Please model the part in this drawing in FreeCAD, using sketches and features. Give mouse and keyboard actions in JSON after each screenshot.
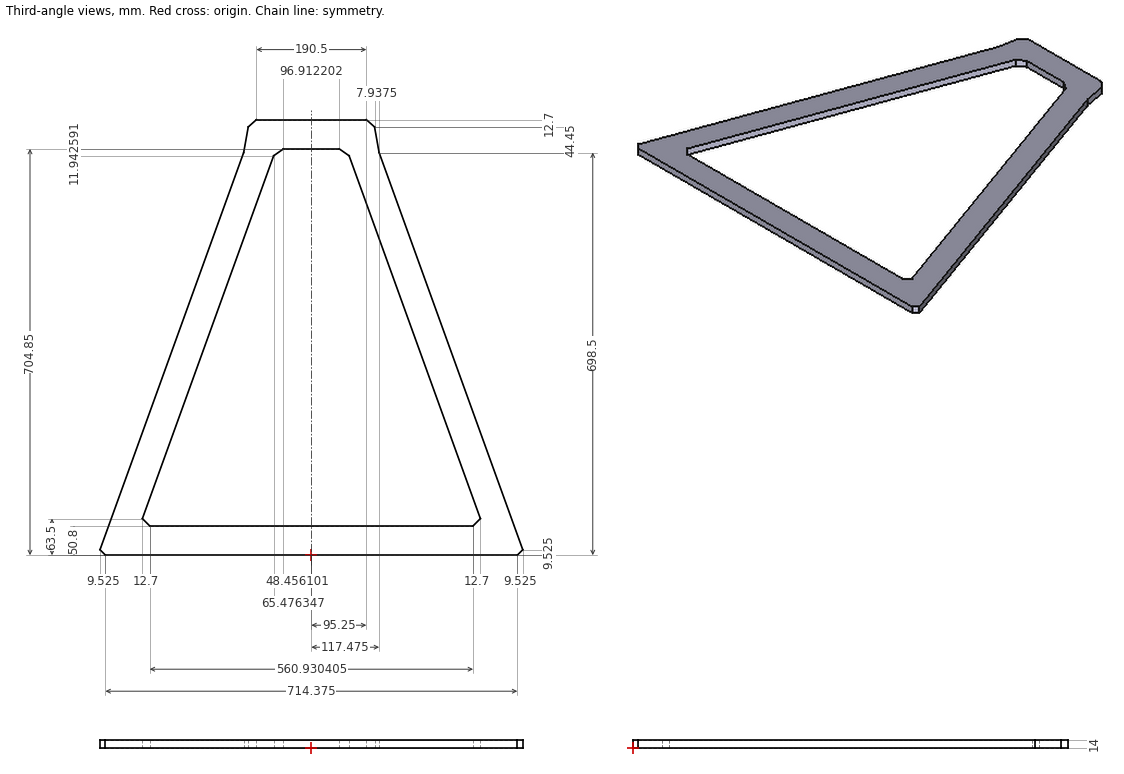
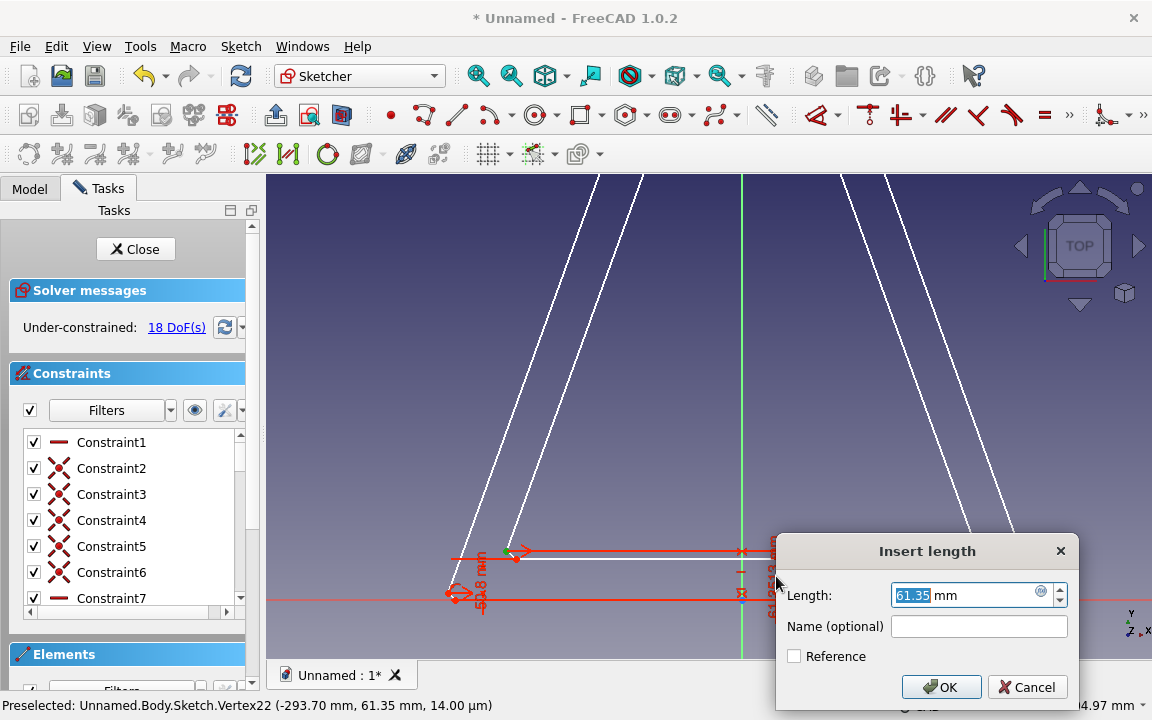
{"action": "type", "text": "63.5"}
{"action": "key", "text": "Return"}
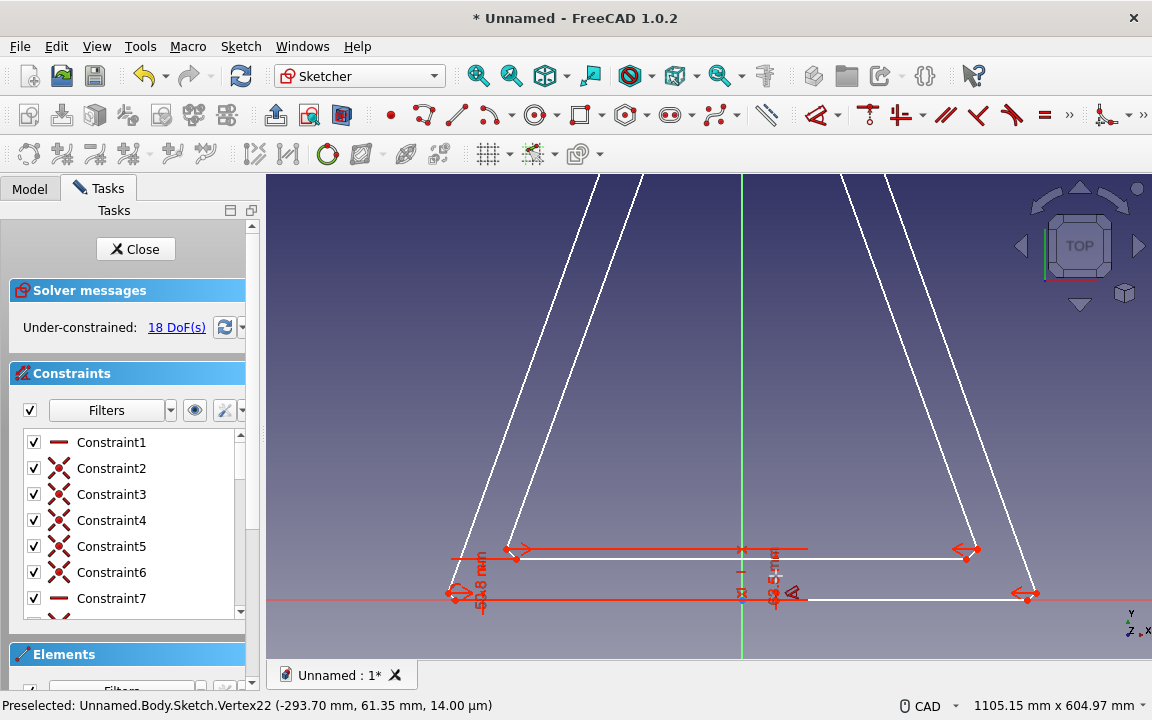
{"action": "scroll", "coordinate": [517, 561], "scroll_direction": "down", "scroll_amount": 3}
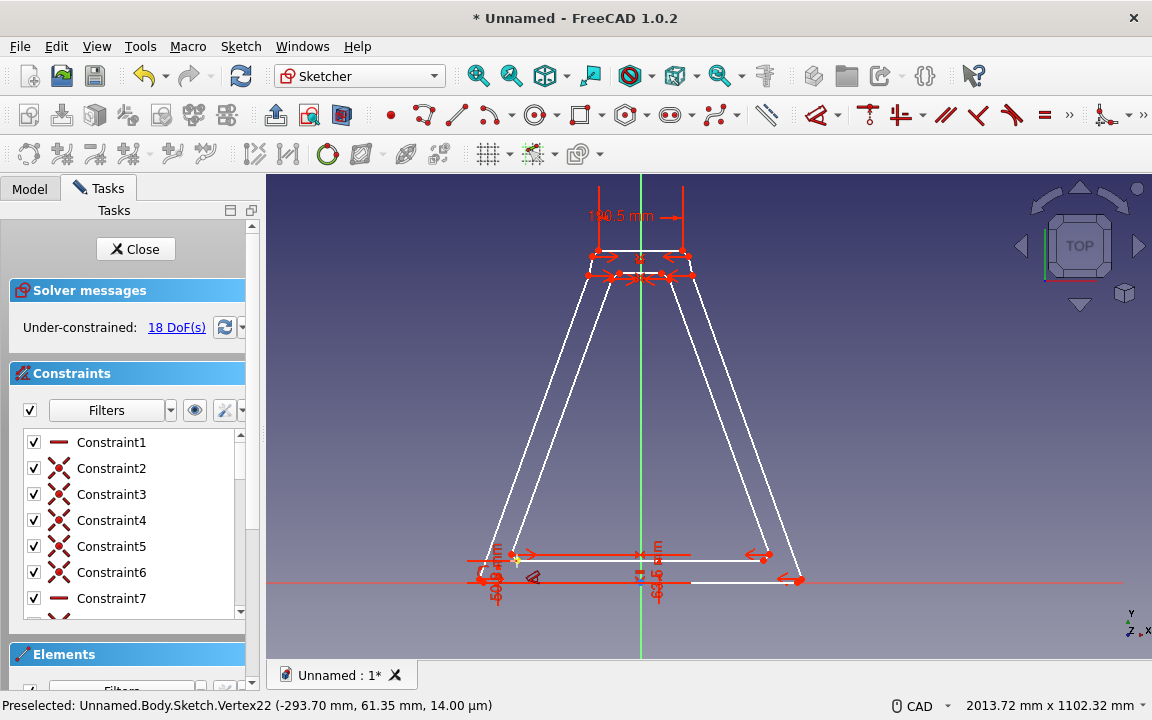
{"action": "scroll", "coordinate": [686, 254], "scroll_direction": "up", "scroll_amount": 10}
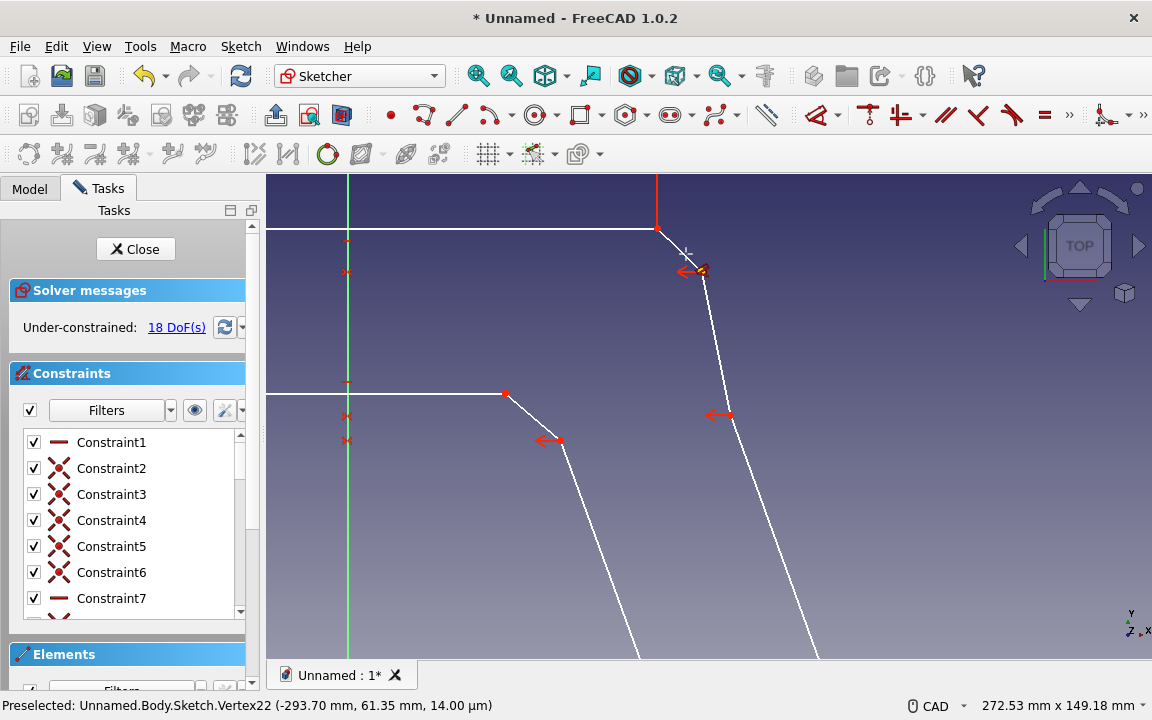
{"action": "left_click", "coordinate": [680, 250]}
{"action": "left_click", "coordinate": [736, 250]}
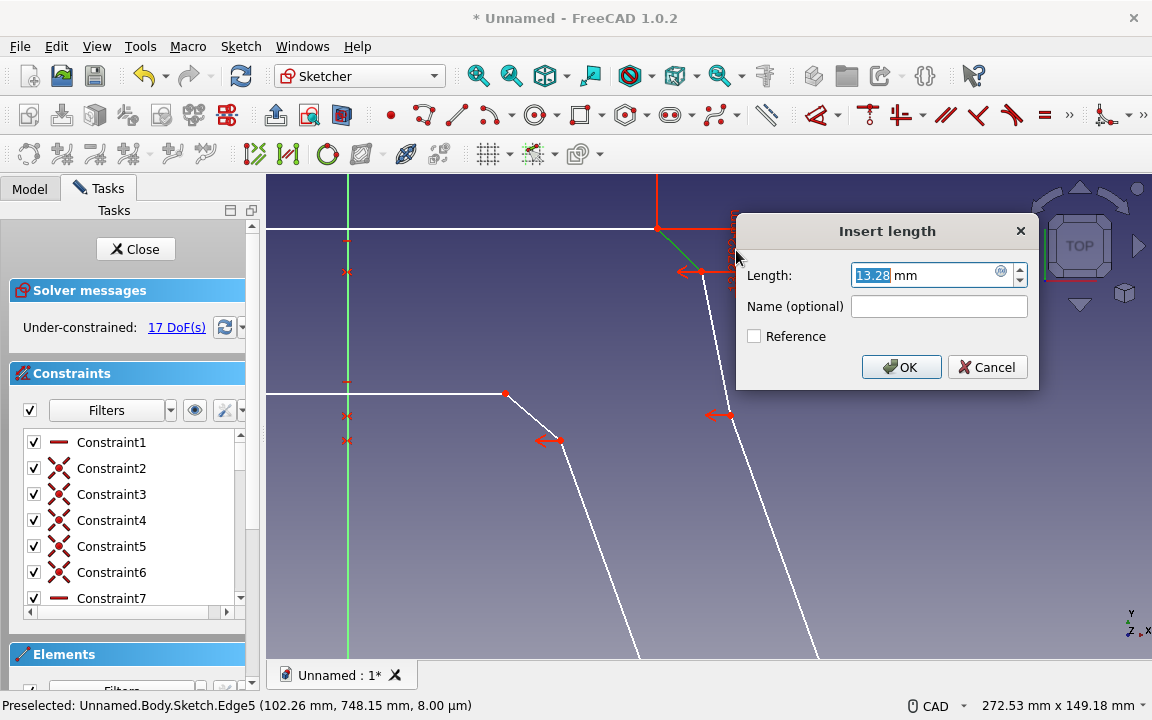
{"action": "type", "text": "12.7"}
{"action": "key", "text": "Return"}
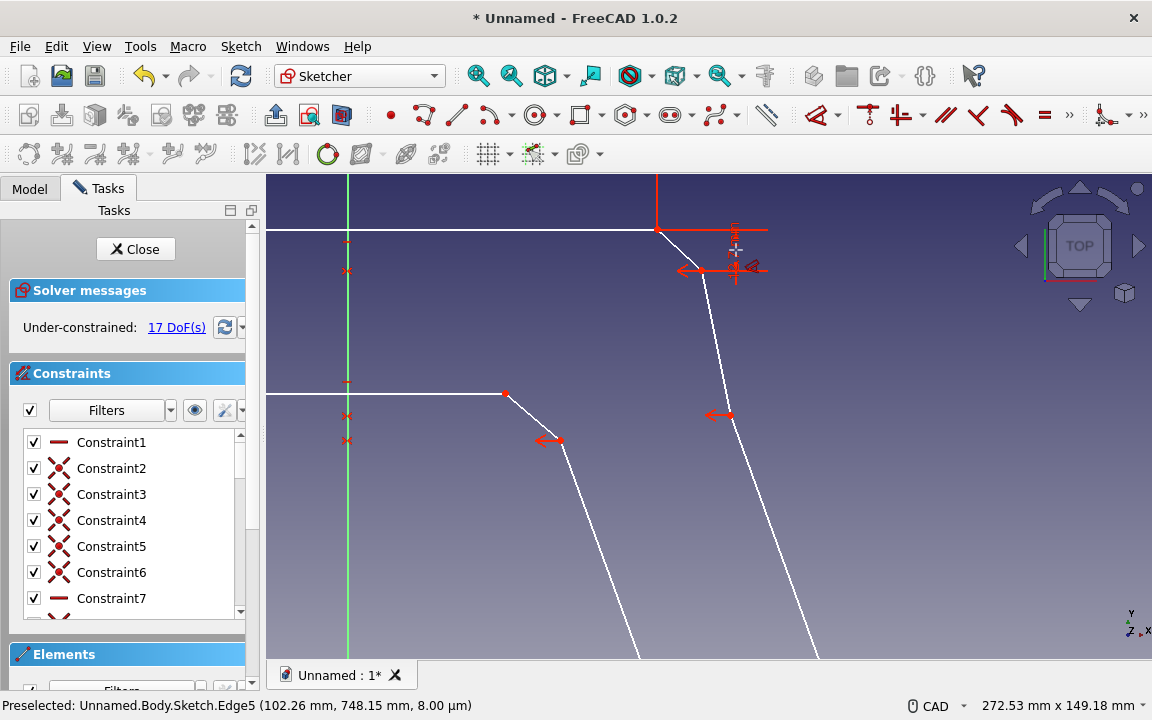
{"action": "scroll", "coordinate": [686, 254], "scroll_direction": "down", "scroll_amount": 10}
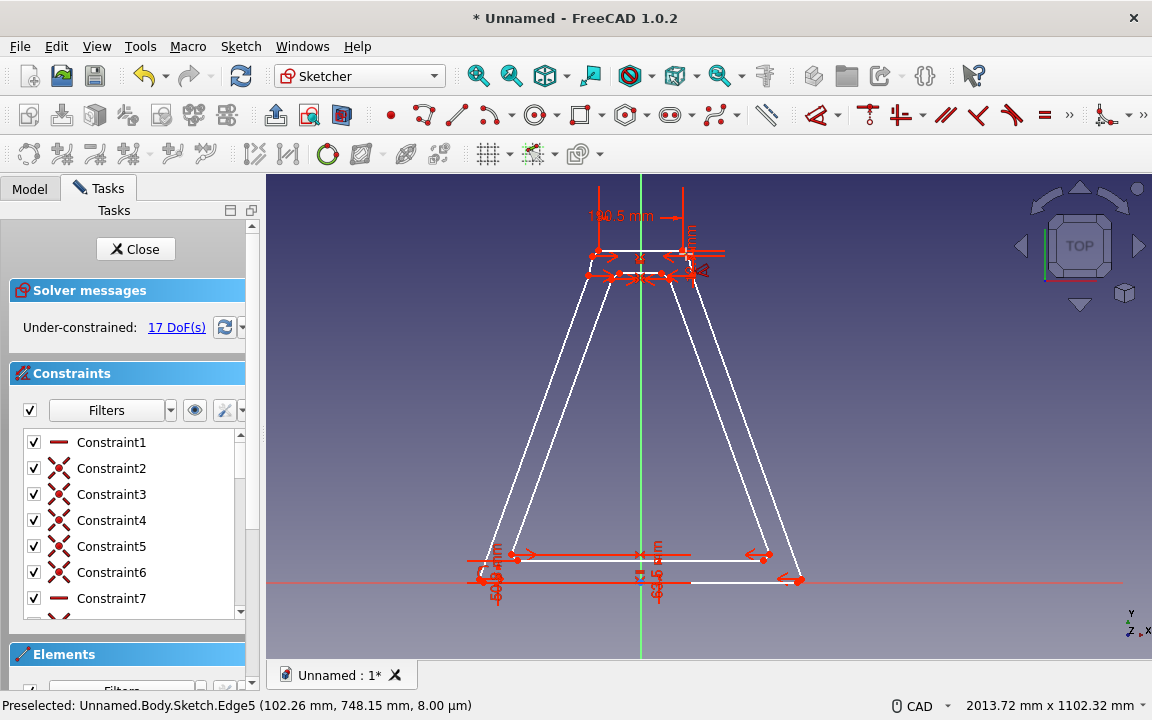
{"action": "scroll", "coordinate": [515, 559], "scroll_direction": "up", "scroll_amount": 10}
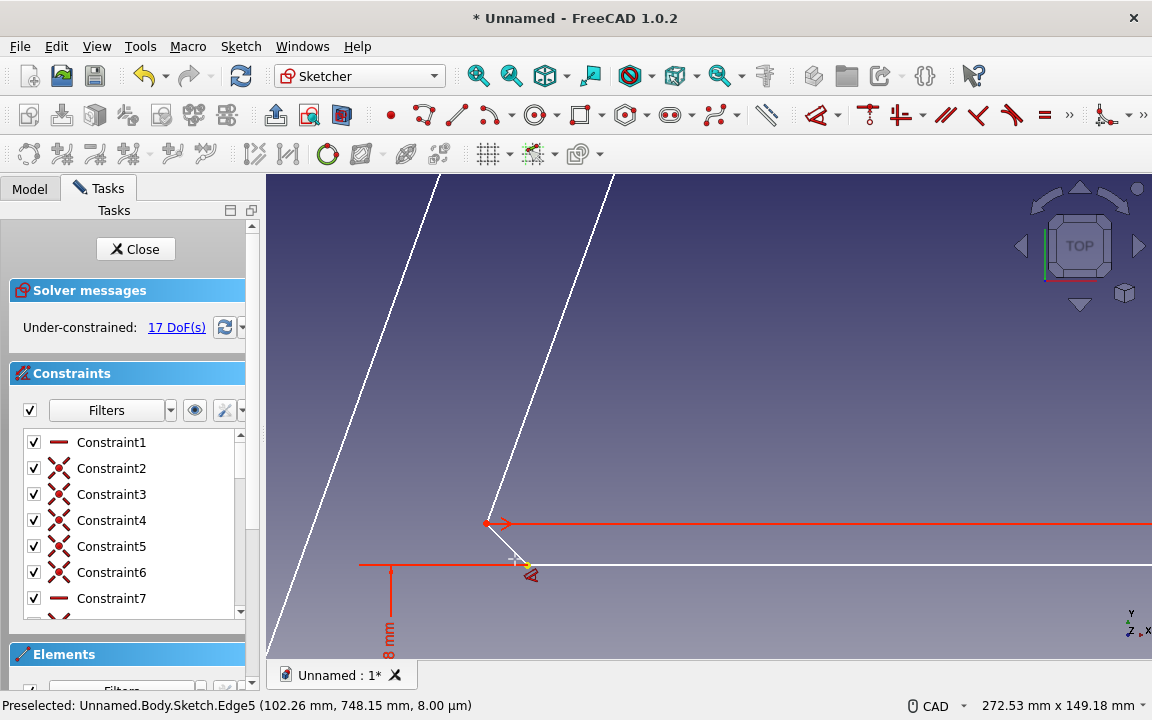
{"action": "left_click", "coordinate": [516, 553]}
{"action": "left_click", "coordinate": [507, 599]}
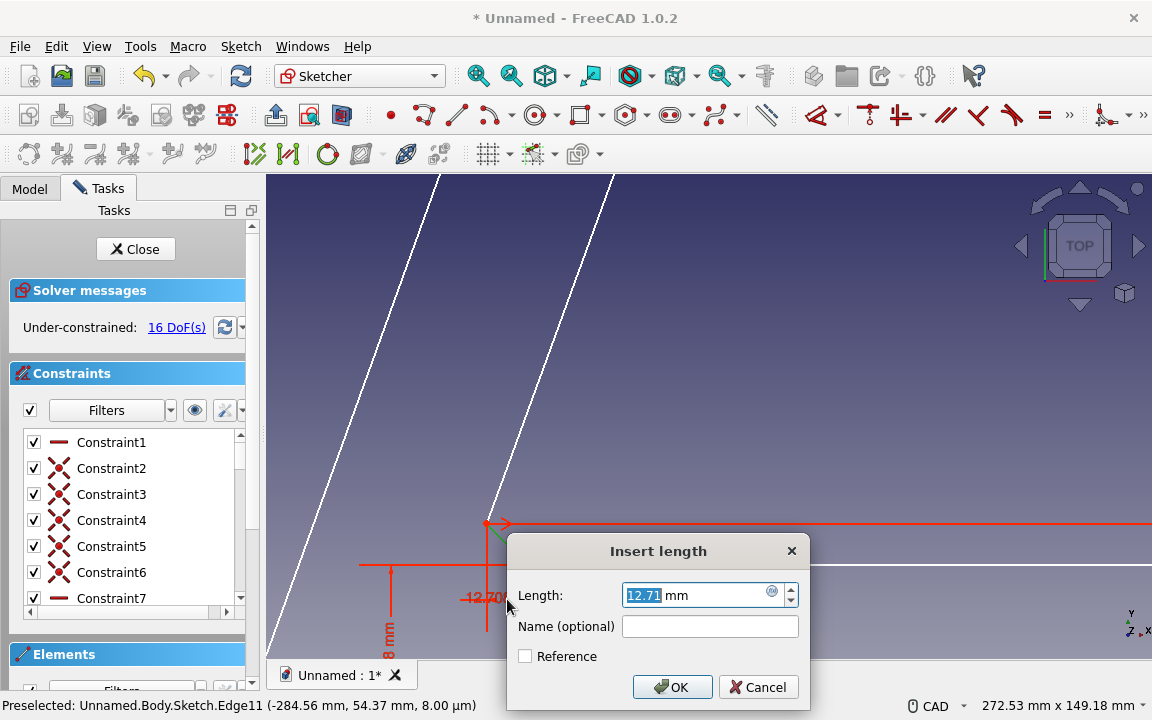
{"action": "type", "text": "12.7"}
{"action": "key", "text": "Return"}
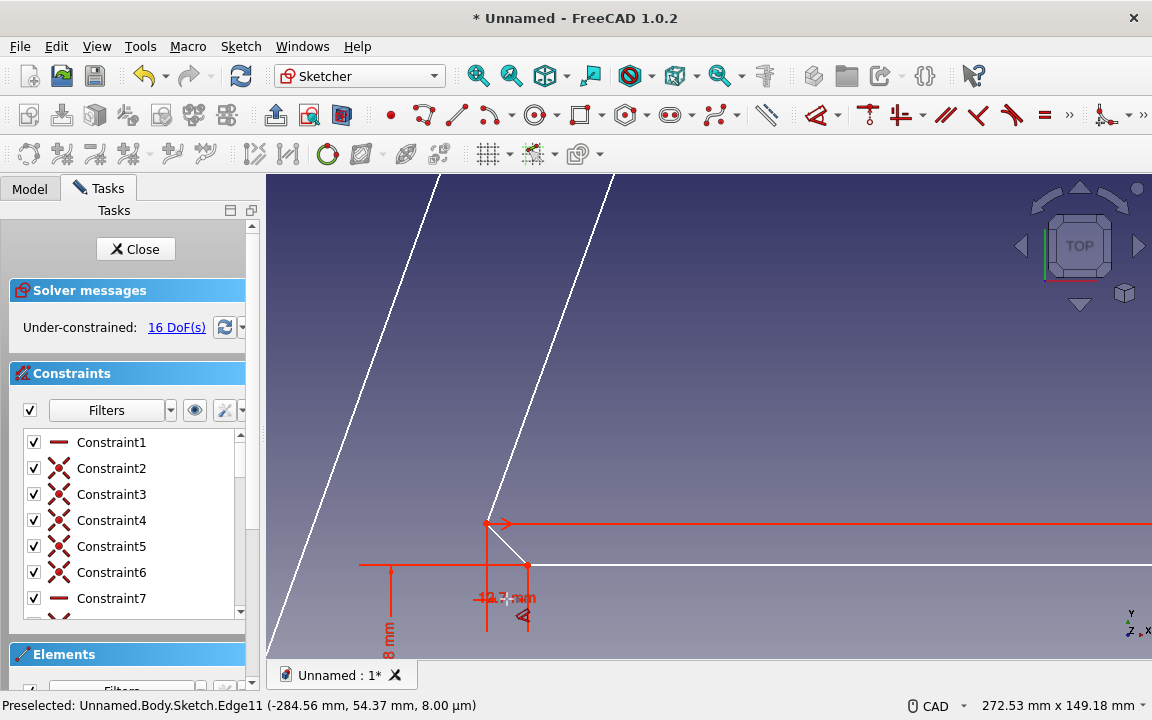
{"action": "scroll", "coordinate": [515, 560], "scroll_direction": "down", "scroll_amount": 10}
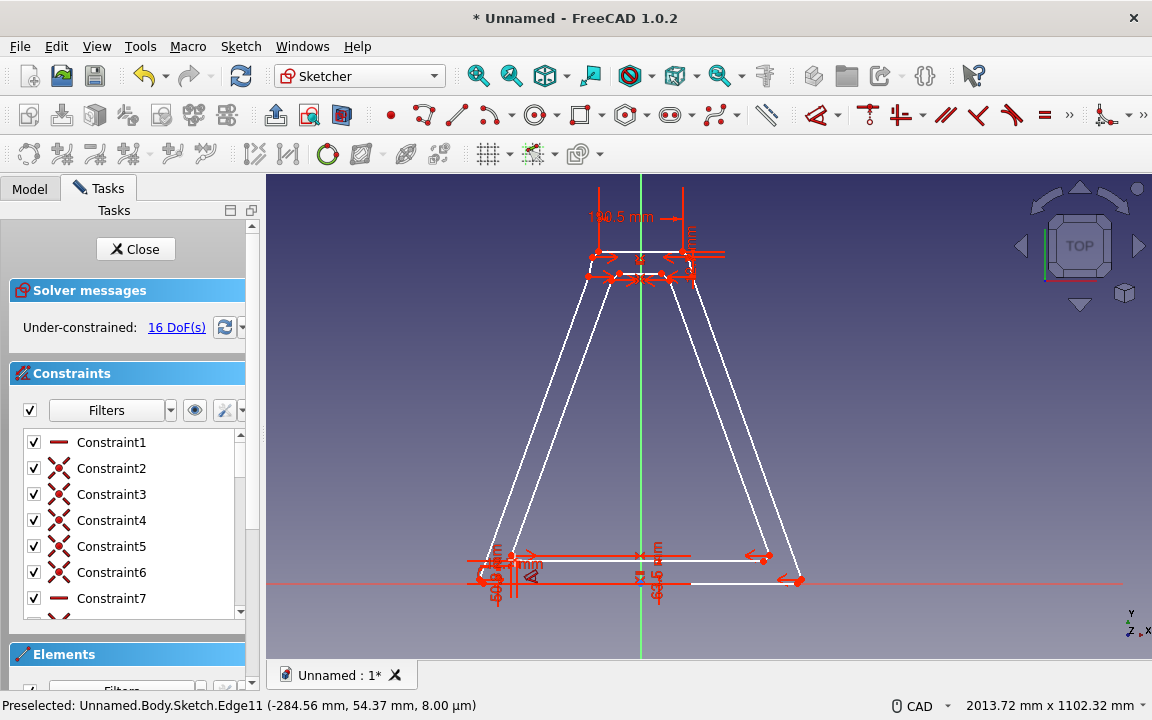
{"action": "scroll", "coordinate": [768, 557], "scroll_direction": "up", "scroll_amount": 10}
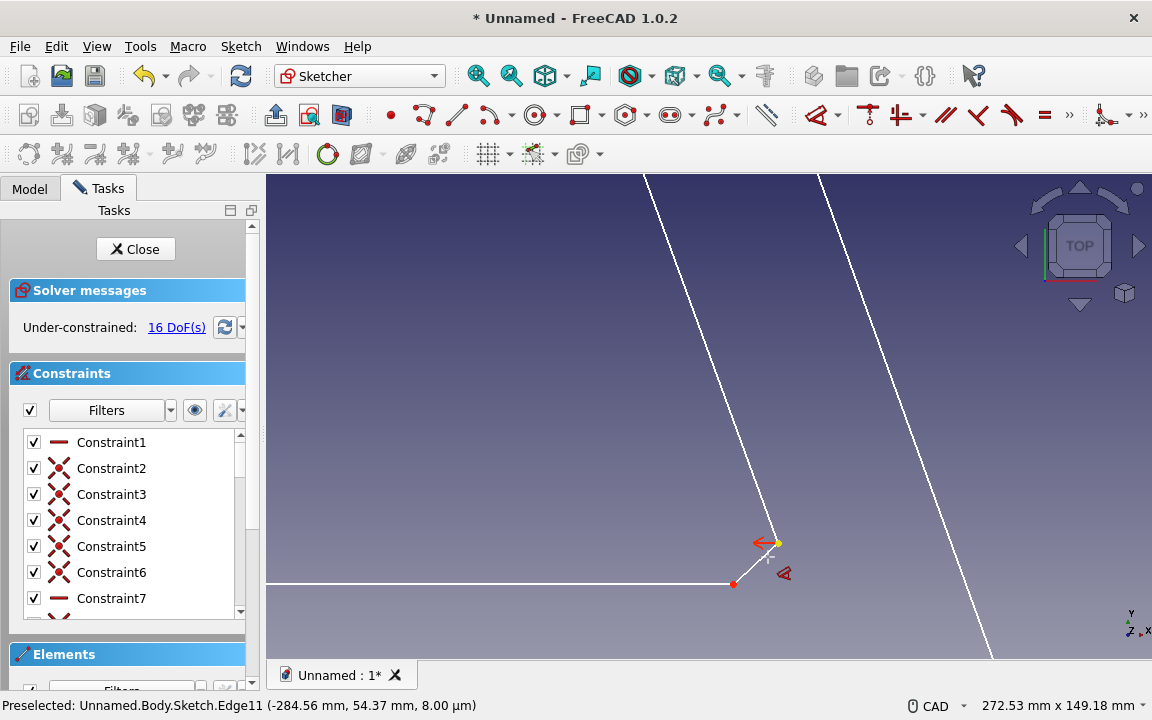
{"action": "left_click", "coordinate": [765, 556]}
{"action": "left_click", "coordinate": [756, 618]}